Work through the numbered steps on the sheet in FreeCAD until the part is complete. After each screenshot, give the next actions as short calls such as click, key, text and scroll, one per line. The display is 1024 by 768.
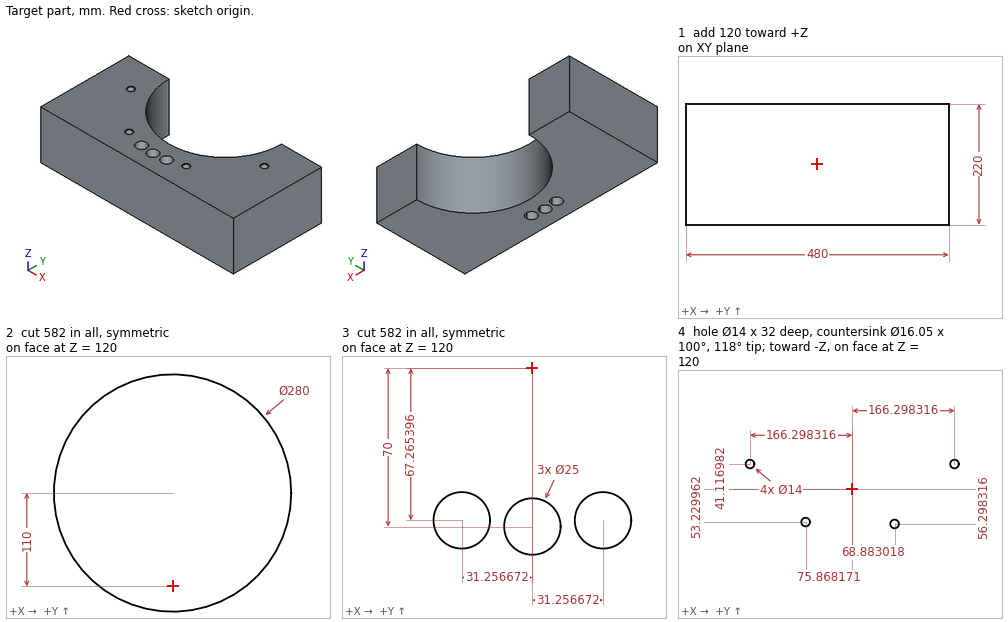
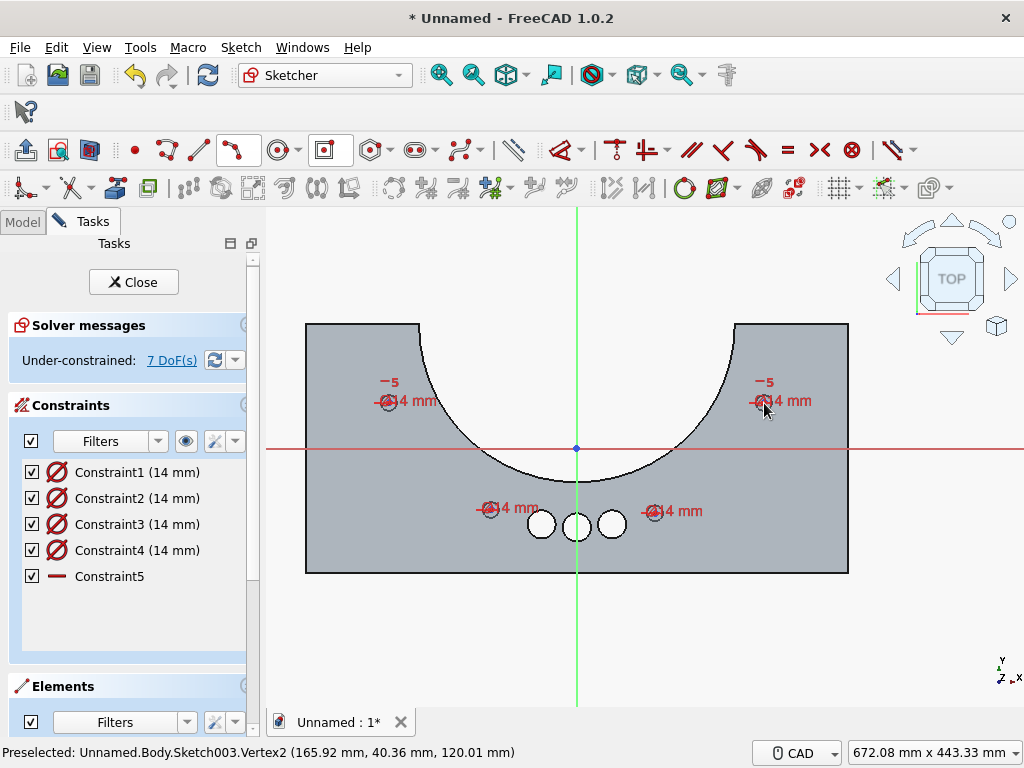
key(d)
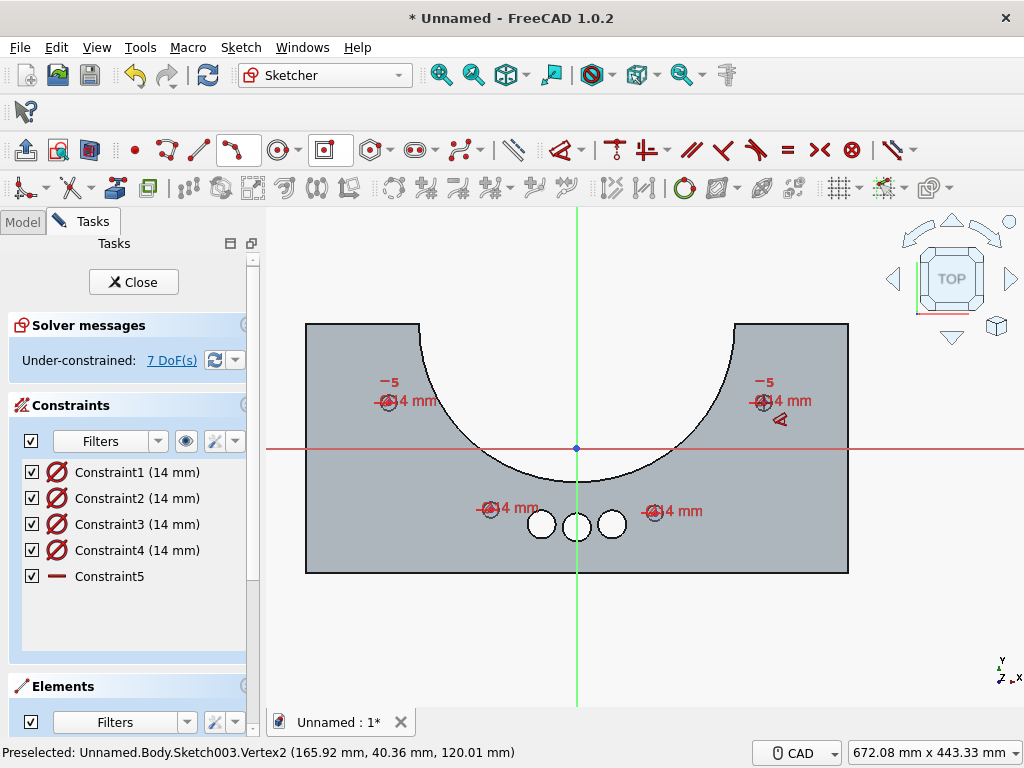
click(389, 403)
click(355, 426)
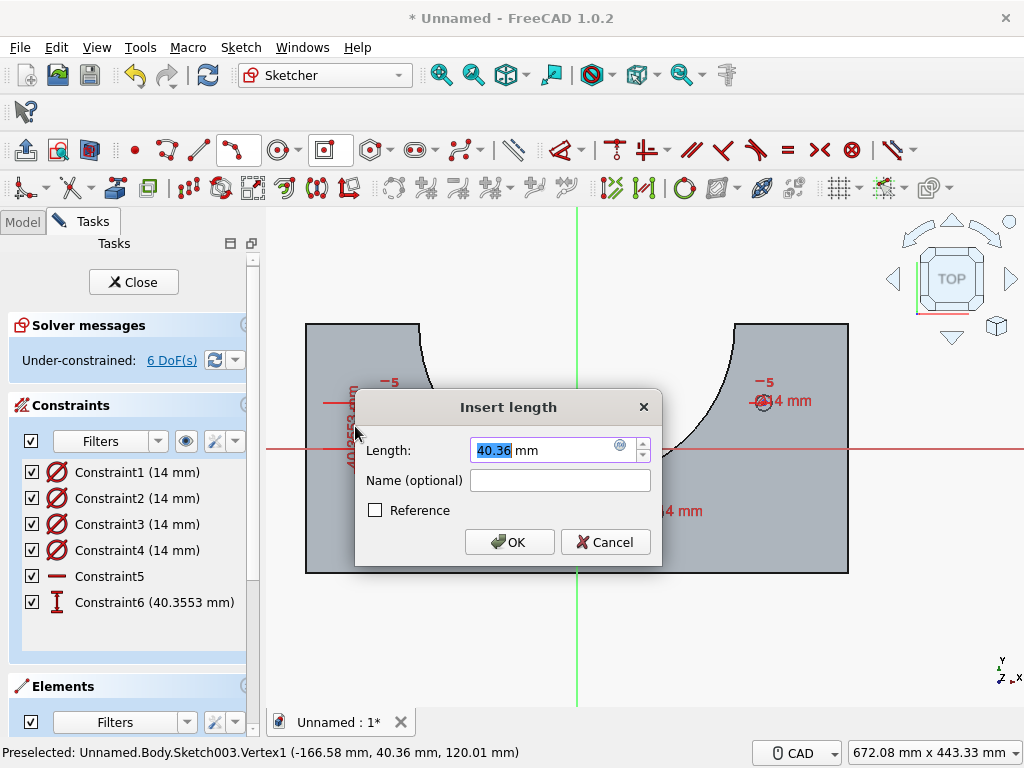
text(41.116982)
key(Return)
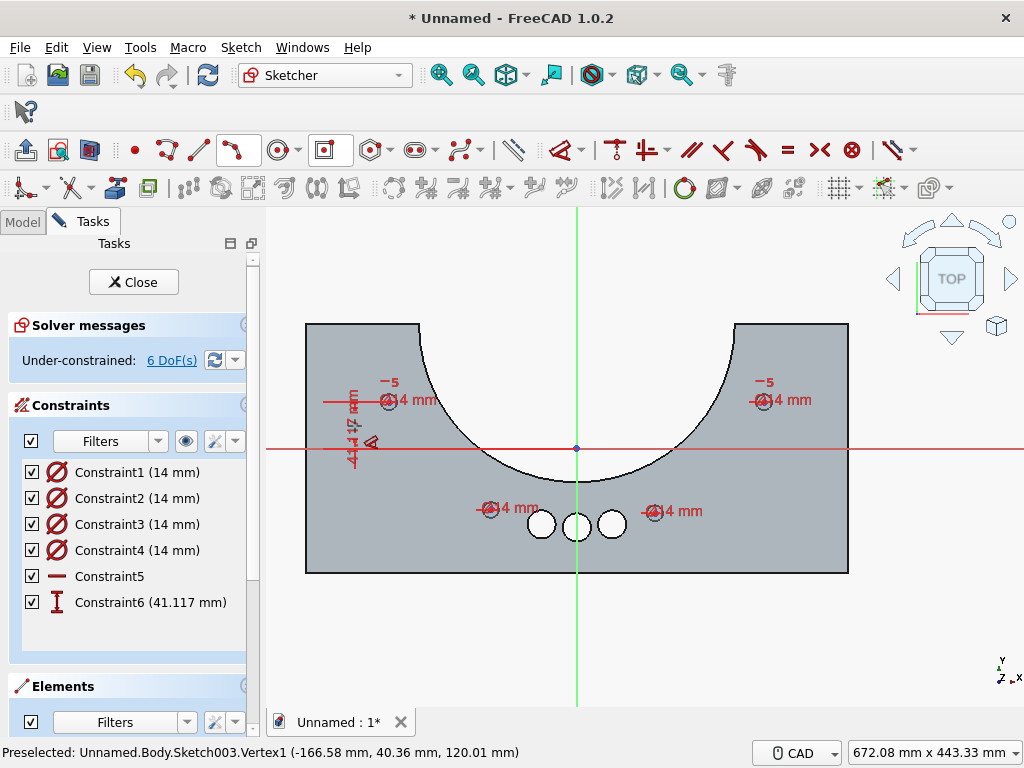
click(655, 513)
click(616, 547)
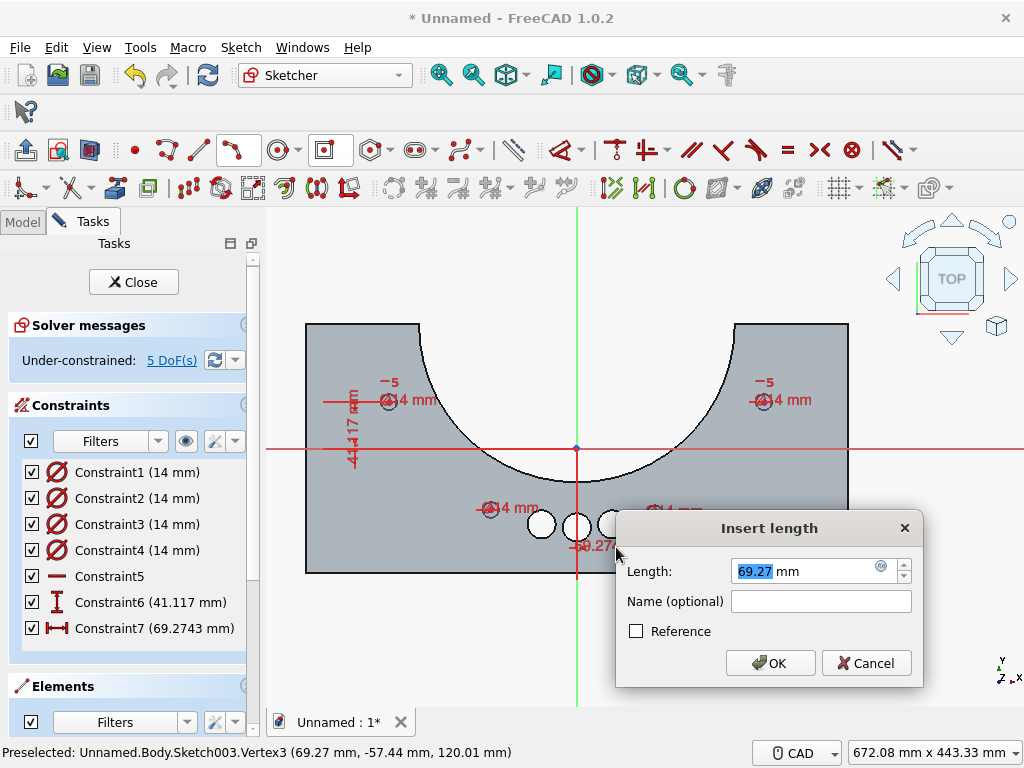
text(68.883018)
key(Return)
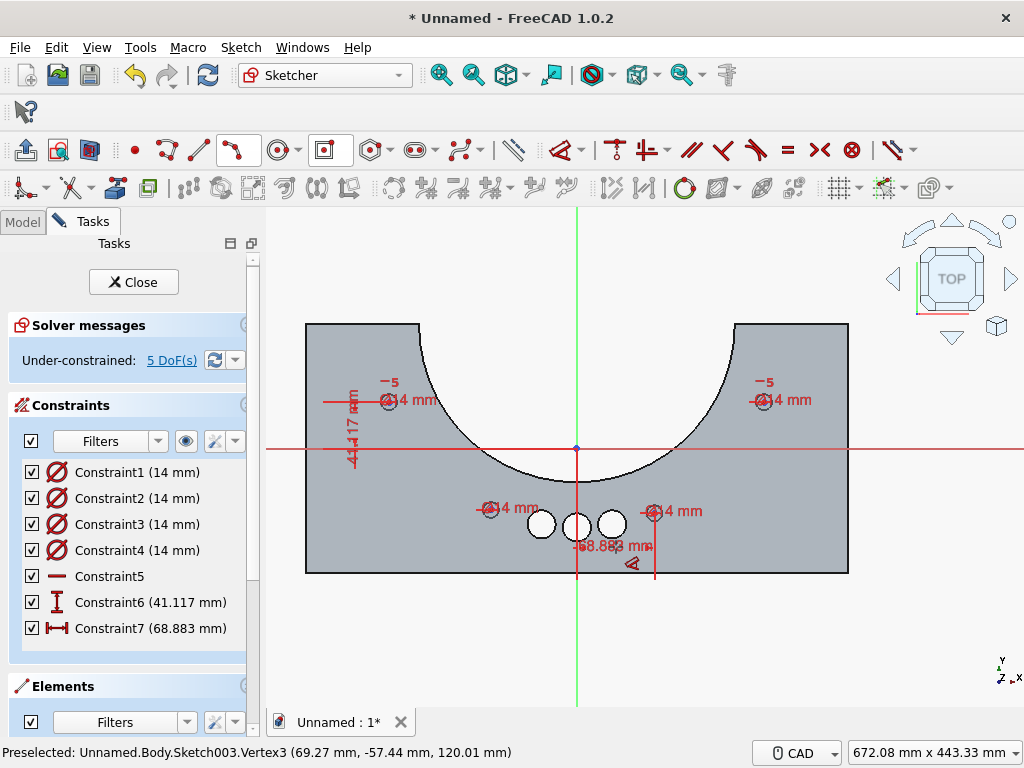
click(655, 513)
click(689, 481)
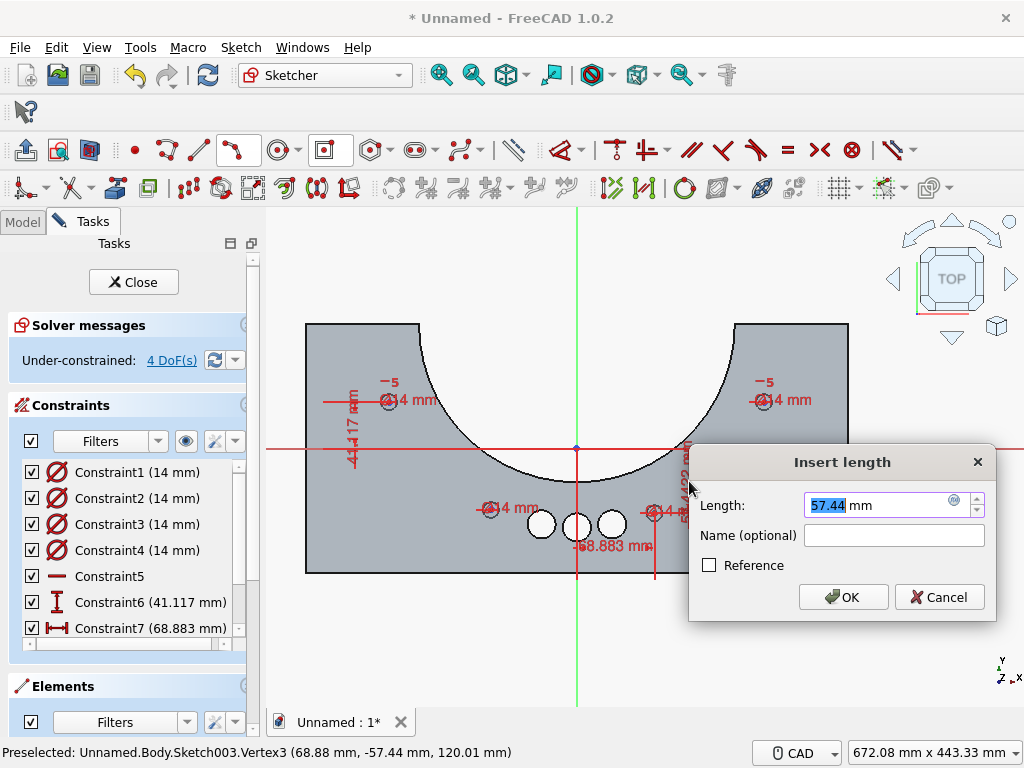
text(56.298316)
key(Return)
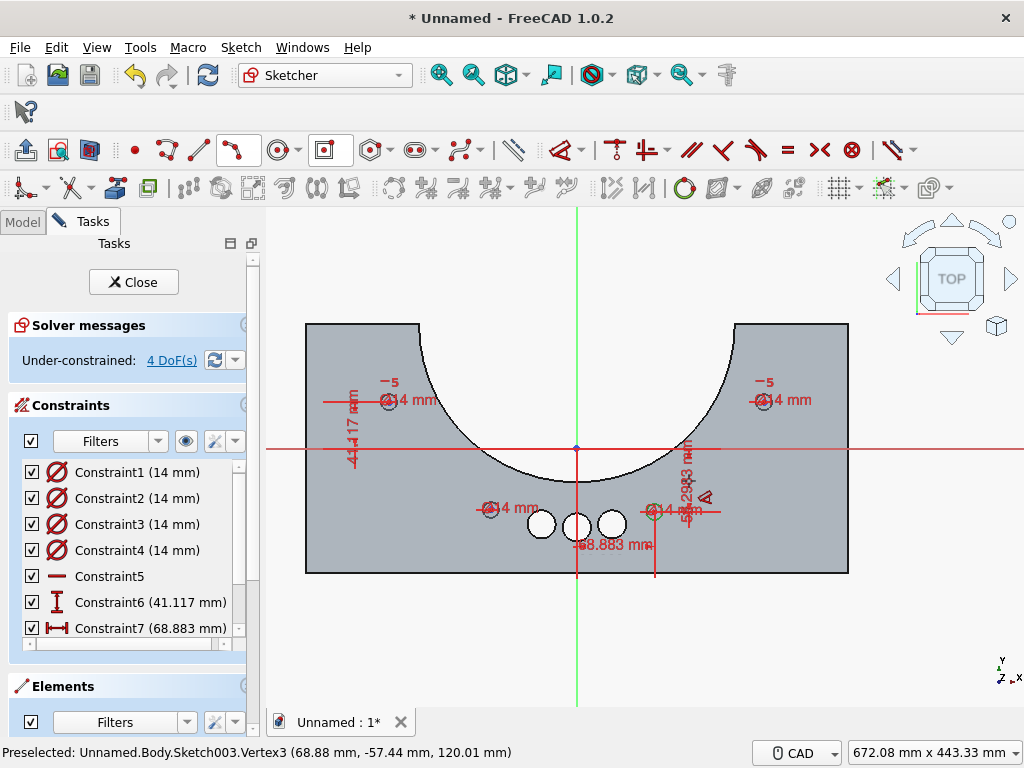
click(491, 510)
click(534, 544)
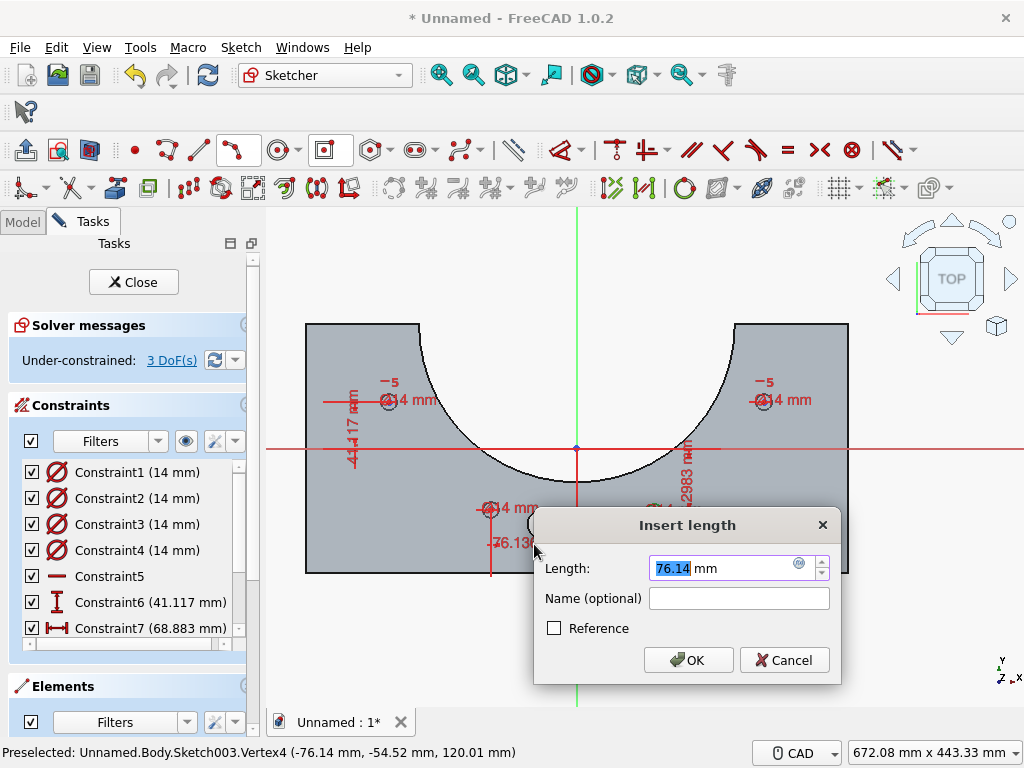
text(75.868171)
key(Return)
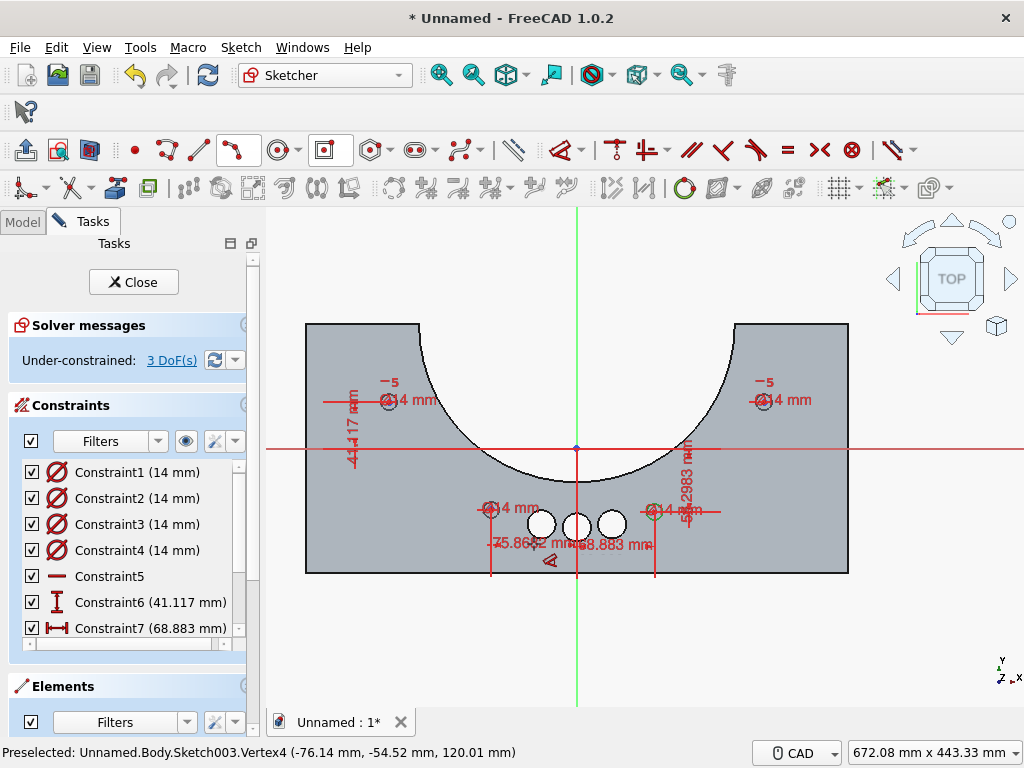
click(491, 510)
click(457, 479)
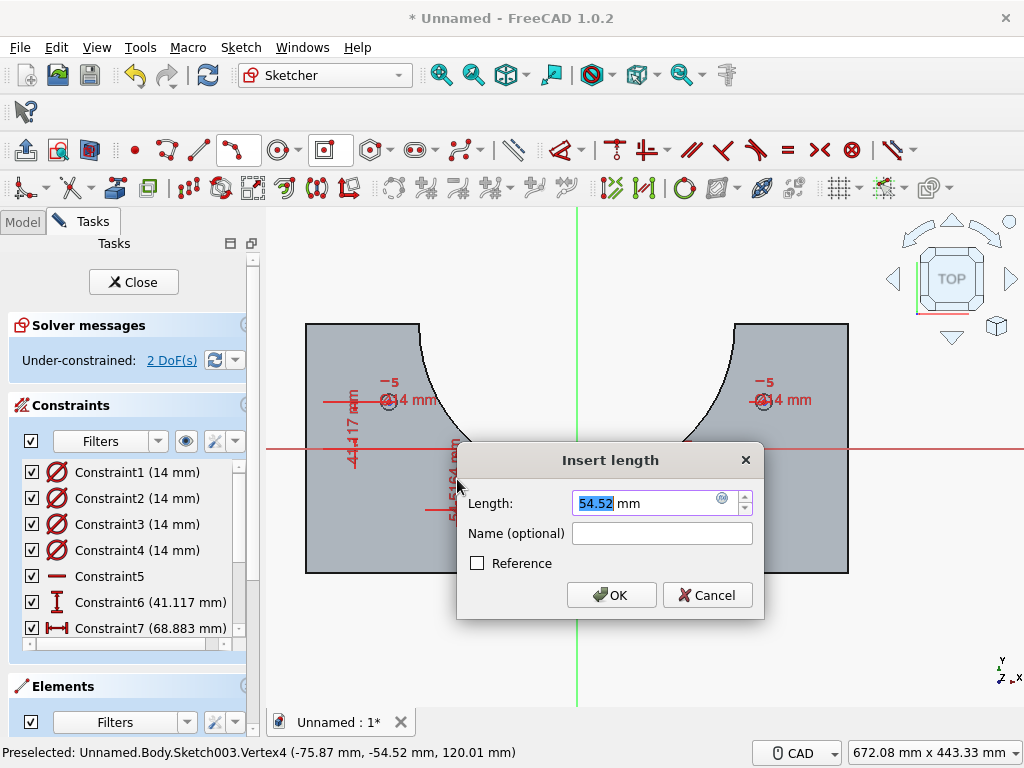
text(53.229962)
key(Return)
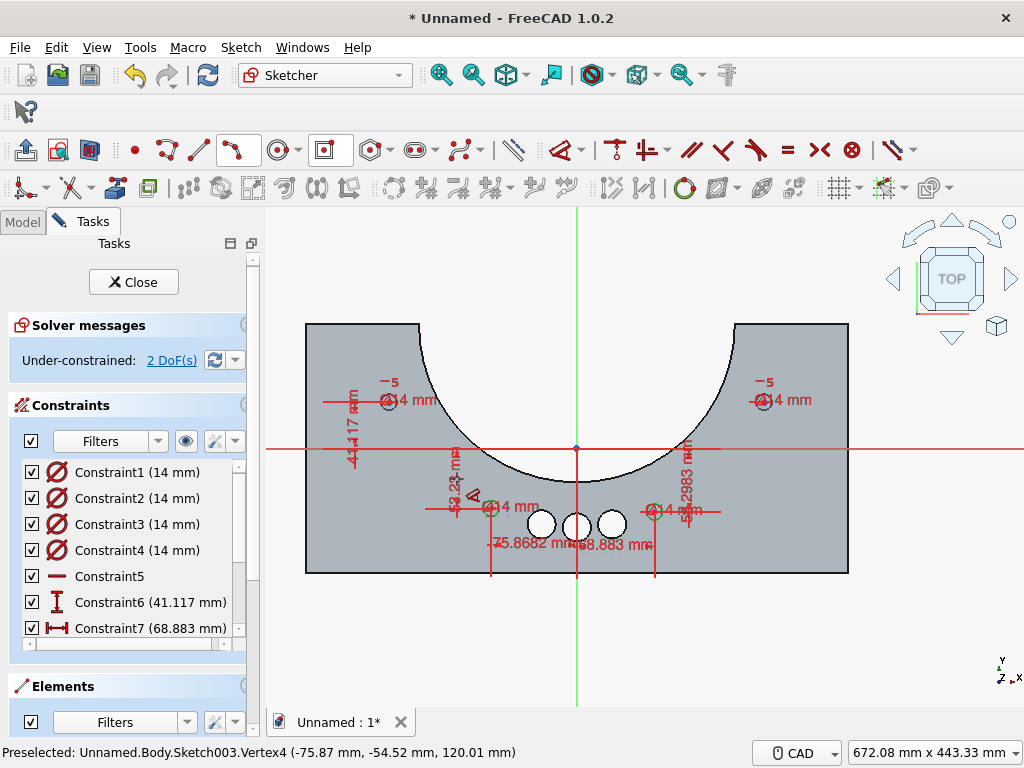
click(389, 402)
click(483, 368)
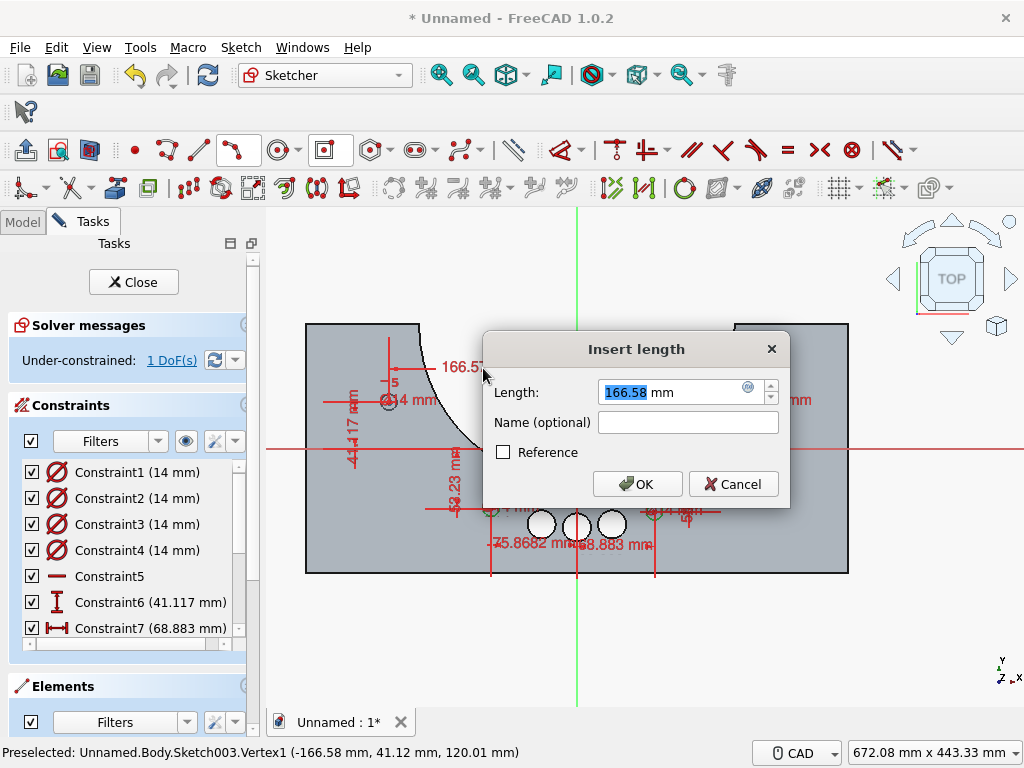
text(166.298316)
key(Return)